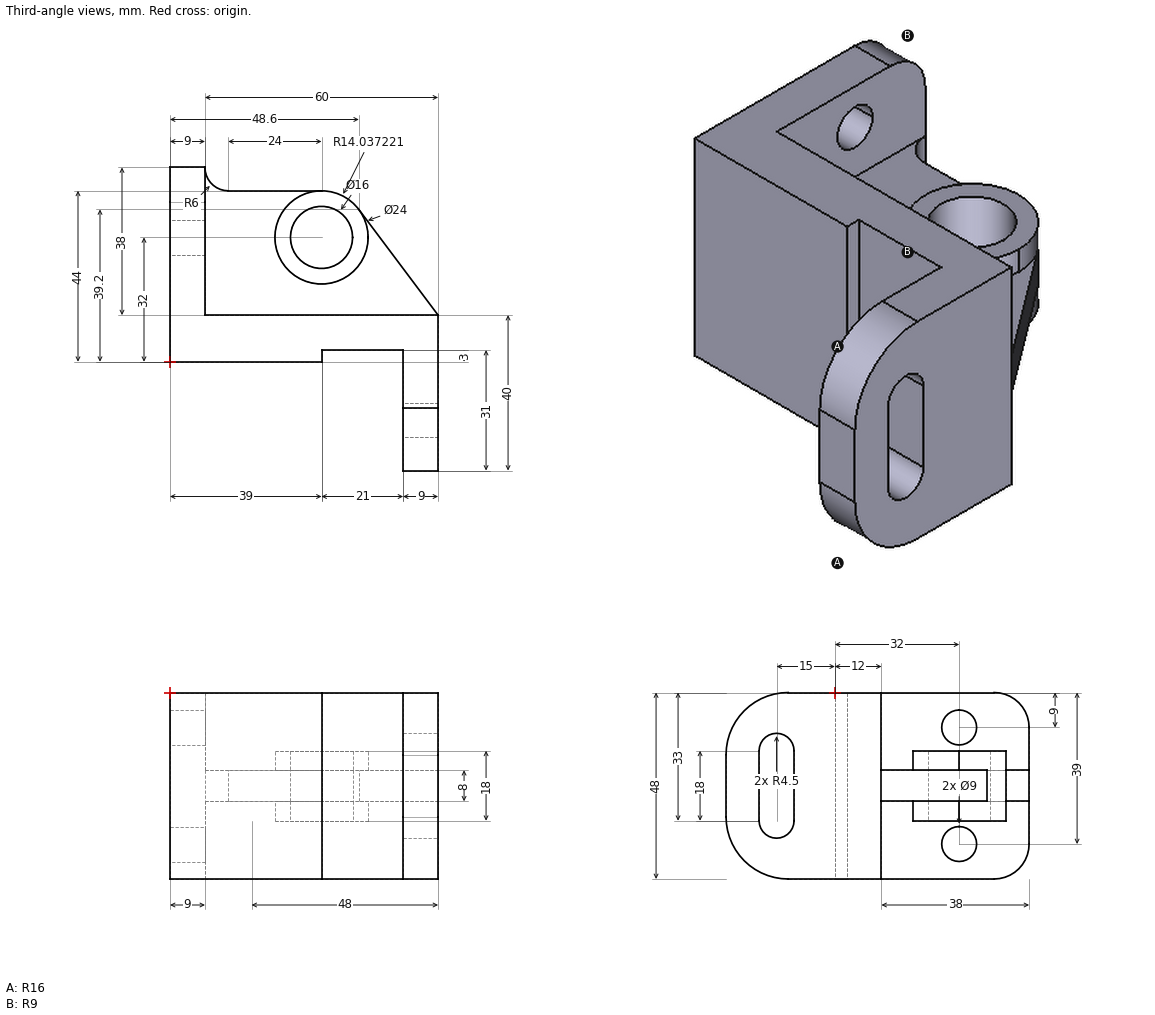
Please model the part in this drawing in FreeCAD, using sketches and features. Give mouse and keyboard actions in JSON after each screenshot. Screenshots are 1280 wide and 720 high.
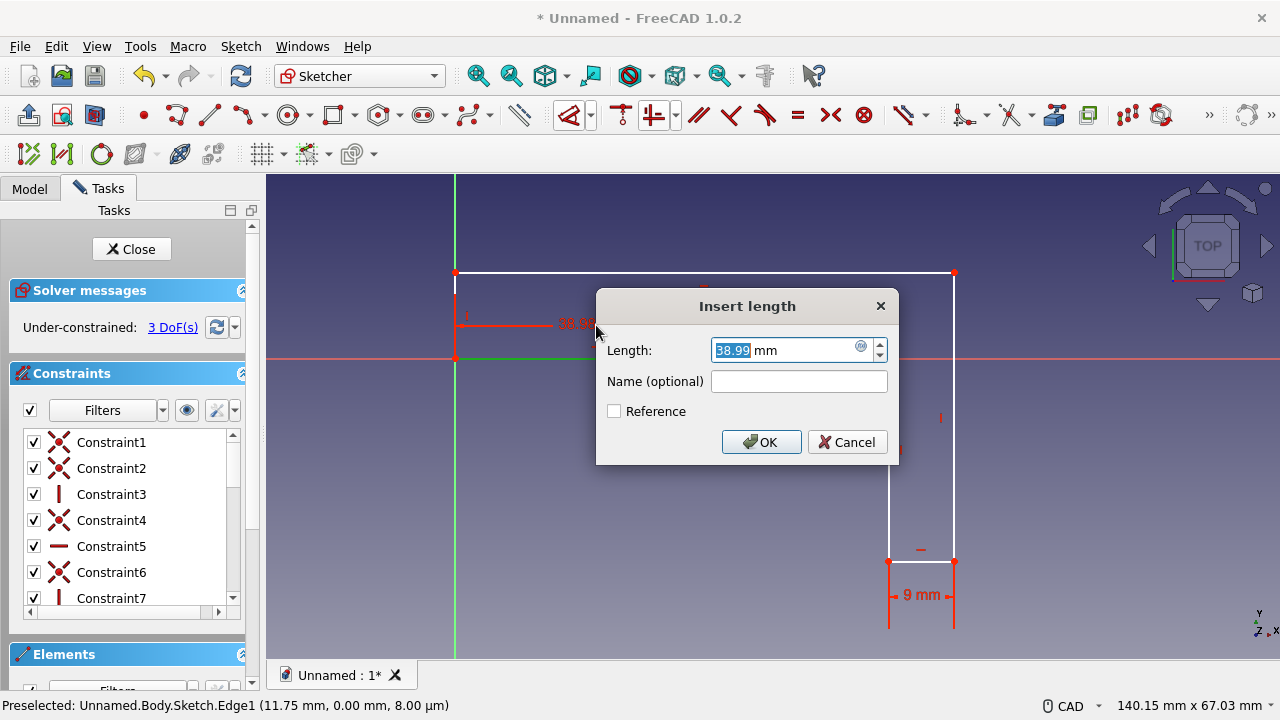
{"action": "type", "text": "39"}
{"action": "key", "text": "Return"}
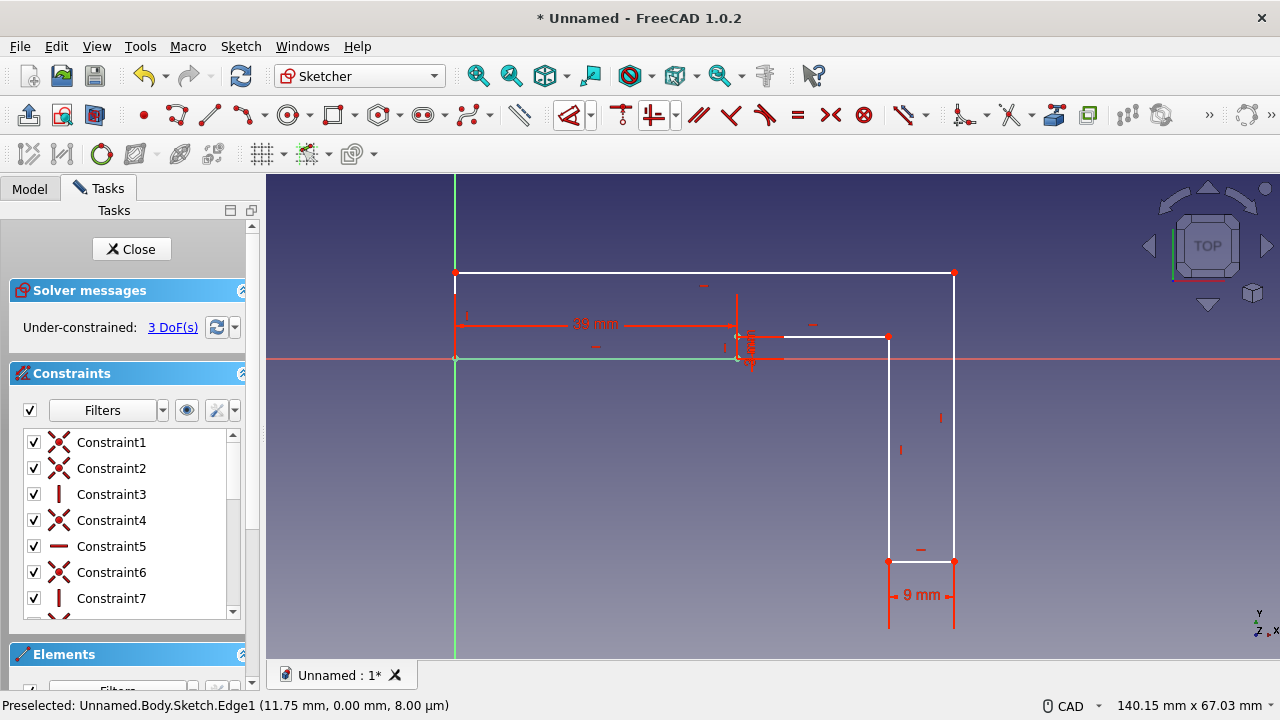
{"action": "left_click", "coordinate": [783, 337]}
{"action": "left_click", "coordinate": [813, 303]}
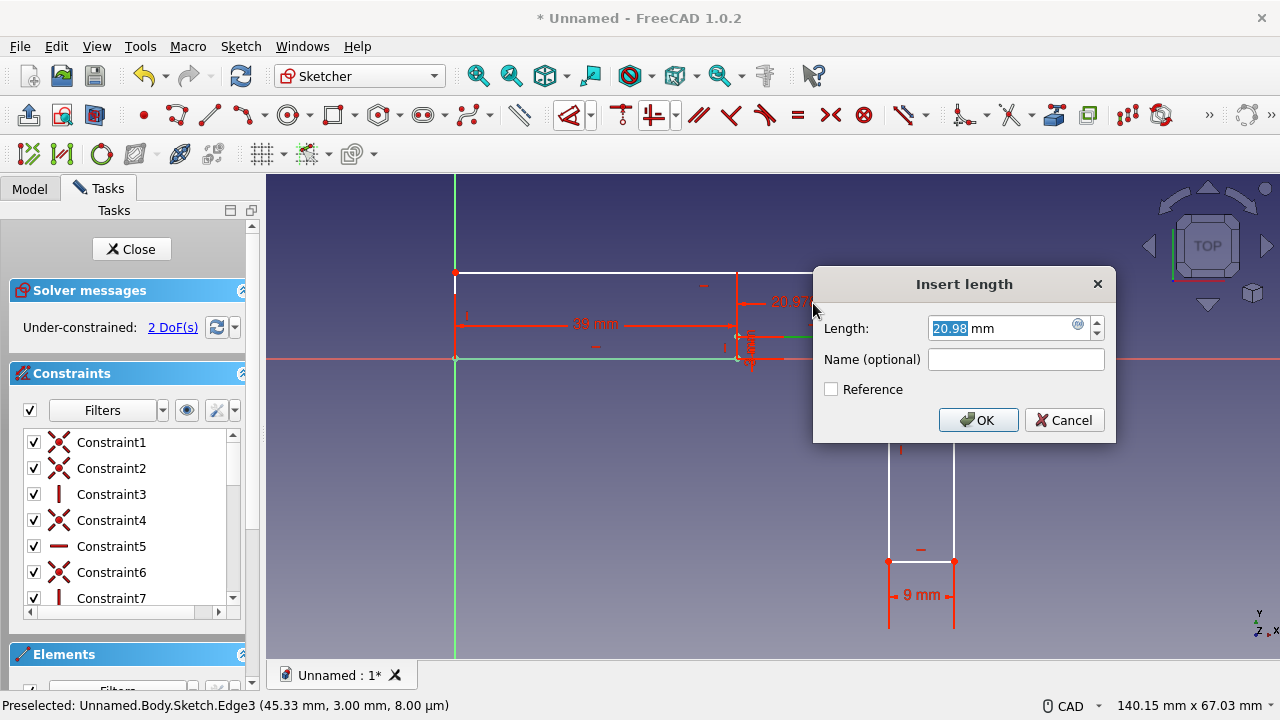
{"action": "type", "text": "21"}
{"action": "key", "text": "Return"}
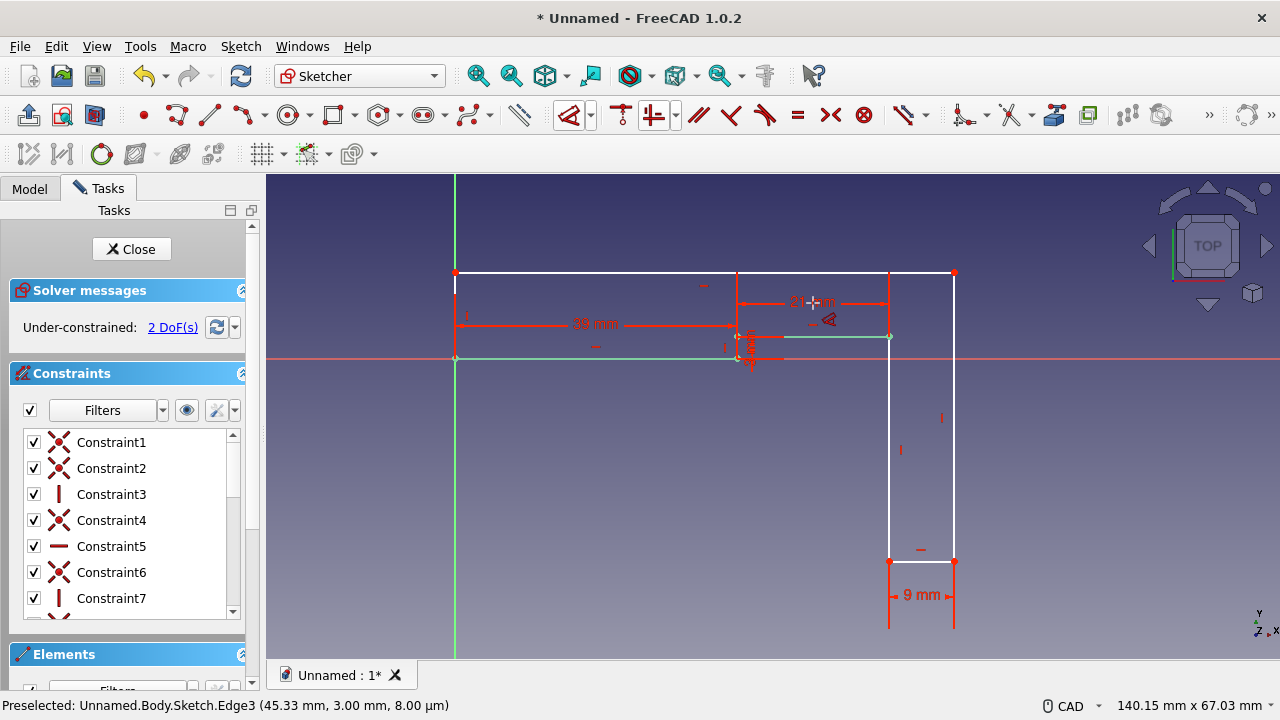
{"action": "left_click", "coordinate": [889, 404]}
{"action": "left_click", "coordinate": [923, 449]}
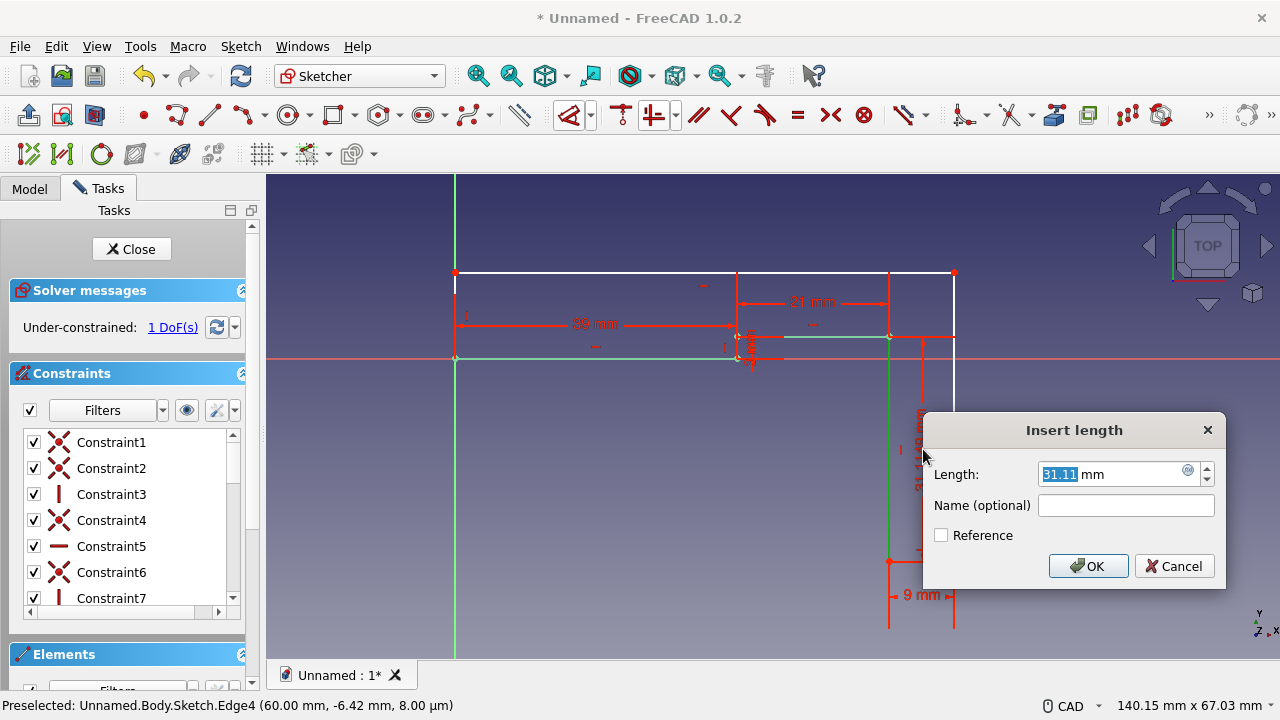
{"action": "type", "text": "31"}
{"action": "key", "text": "Return"}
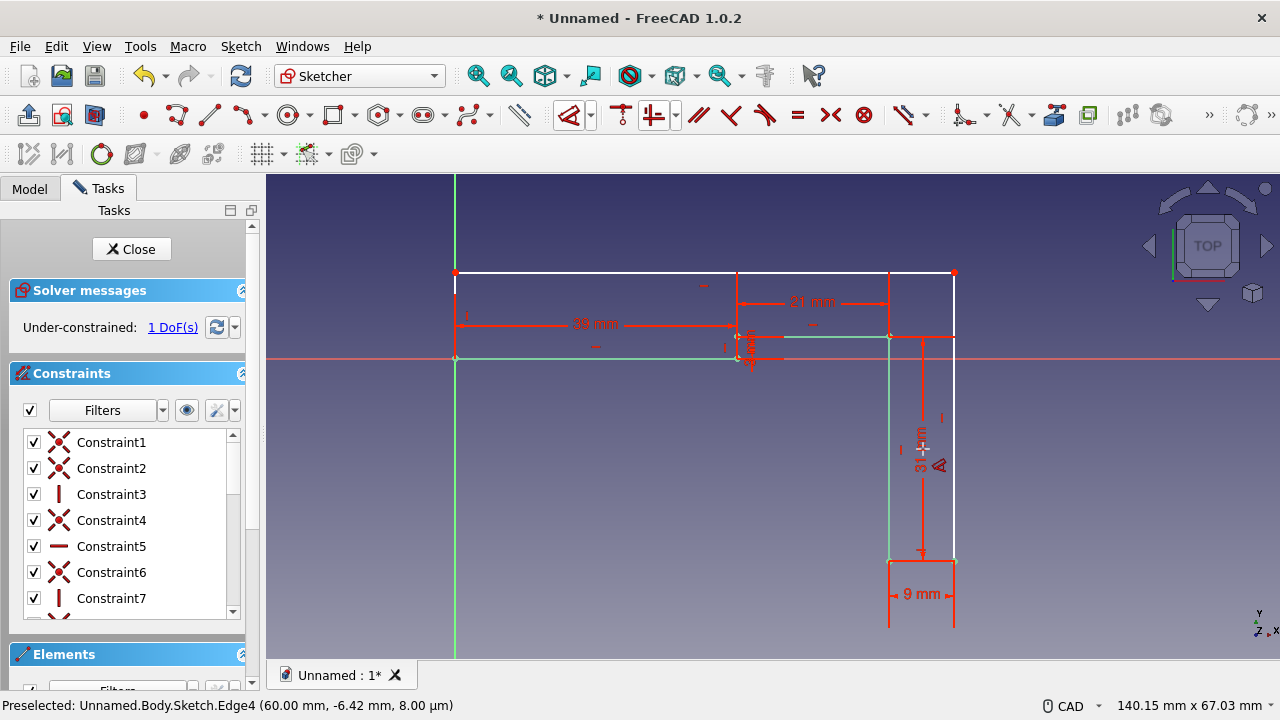
{"action": "left_click", "coordinate": [954, 475]}
{"action": "left_click", "coordinate": [988, 417]}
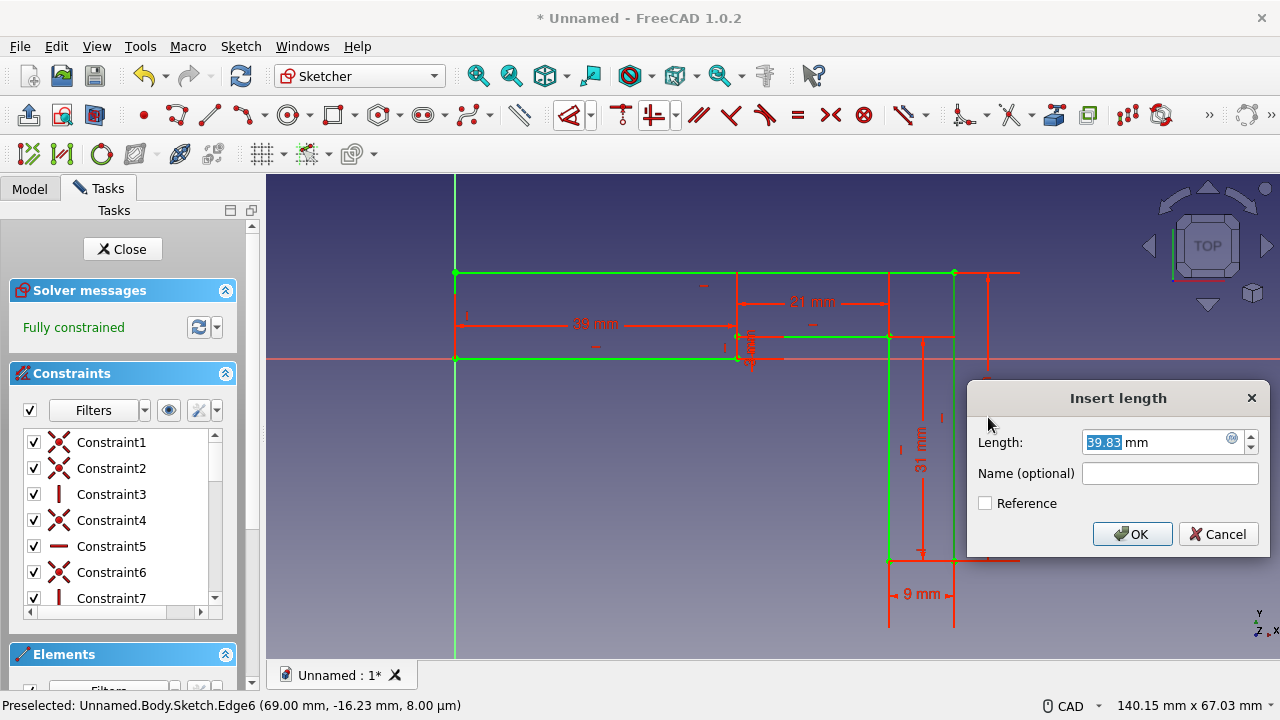
{"action": "type", "text": "40"}
{"action": "key", "text": "Return"}
{"action": "key", "text": "Escape"}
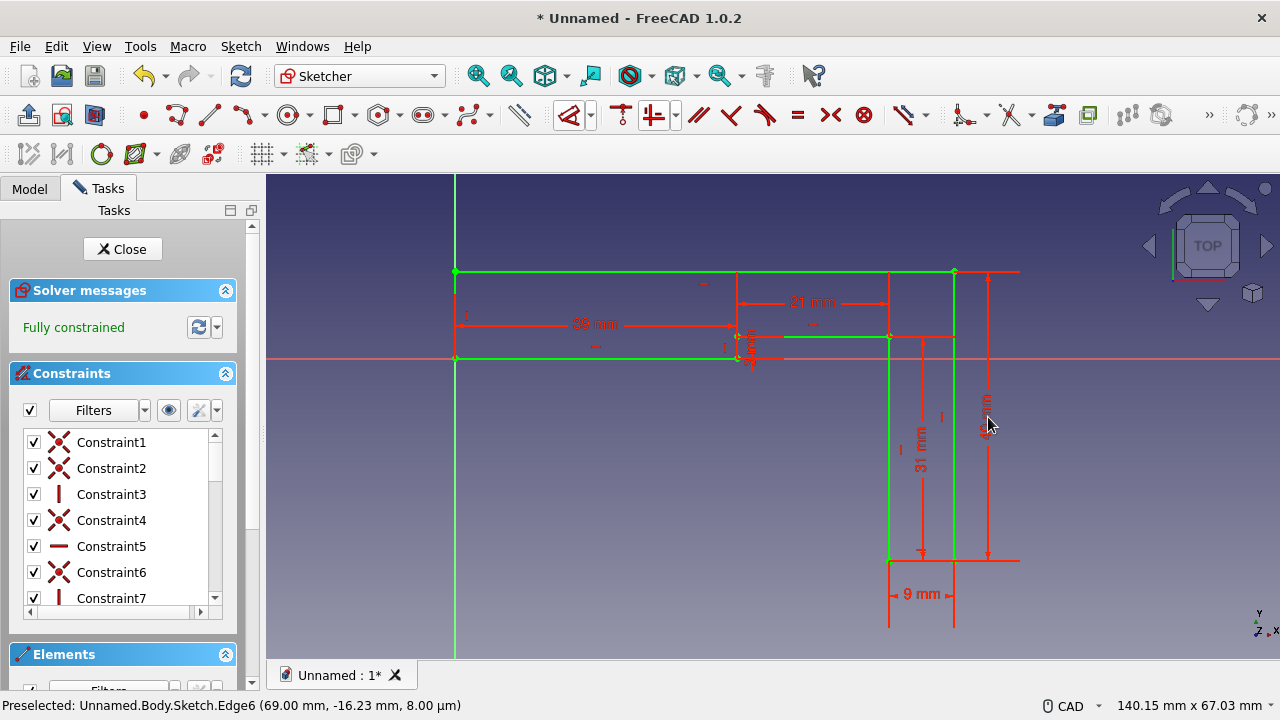
{"action": "left_click", "coordinate": [123, 249]}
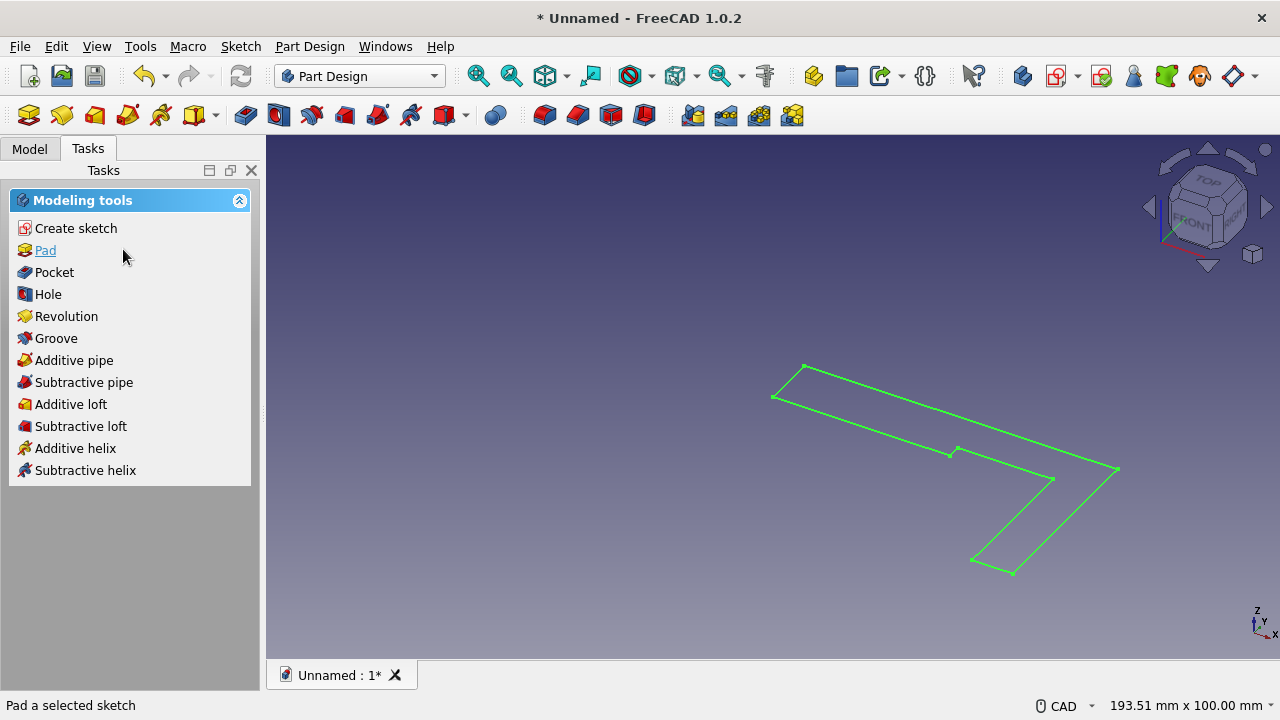
{"action": "left_click", "coordinate": [29, 116]}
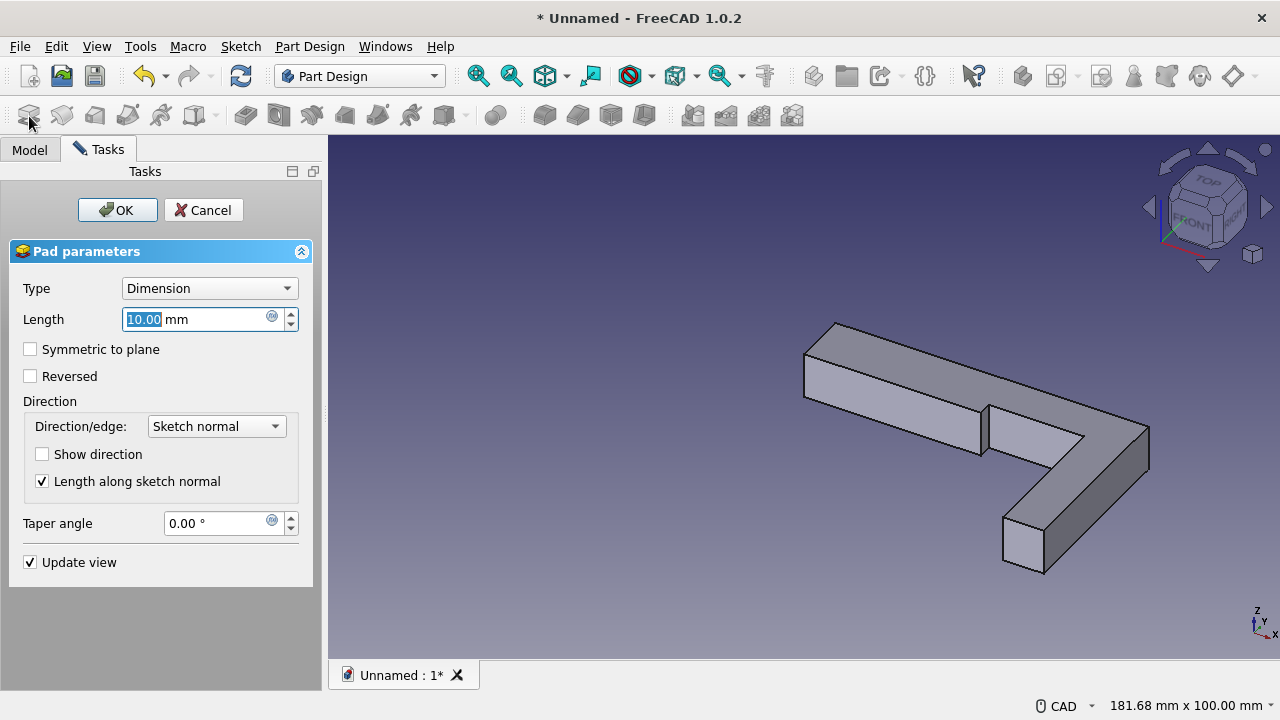
{"action": "type", "text": "48"}
{"action": "key", "text": "Tab"}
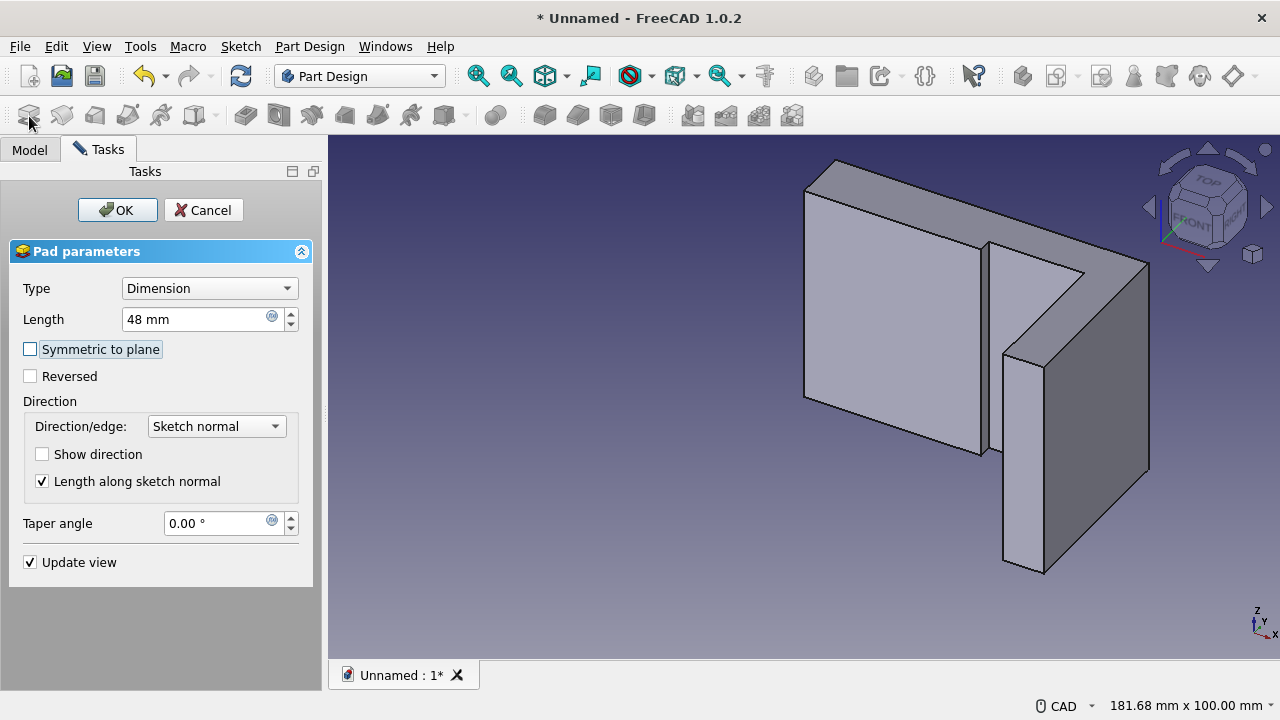
{"action": "left_click", "coordinate": [31, 376]}